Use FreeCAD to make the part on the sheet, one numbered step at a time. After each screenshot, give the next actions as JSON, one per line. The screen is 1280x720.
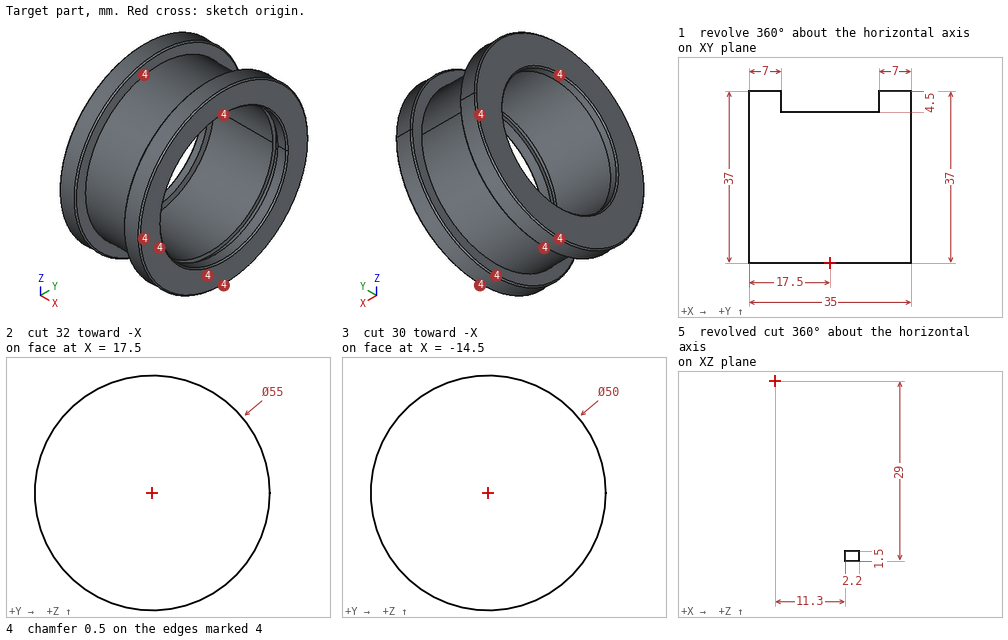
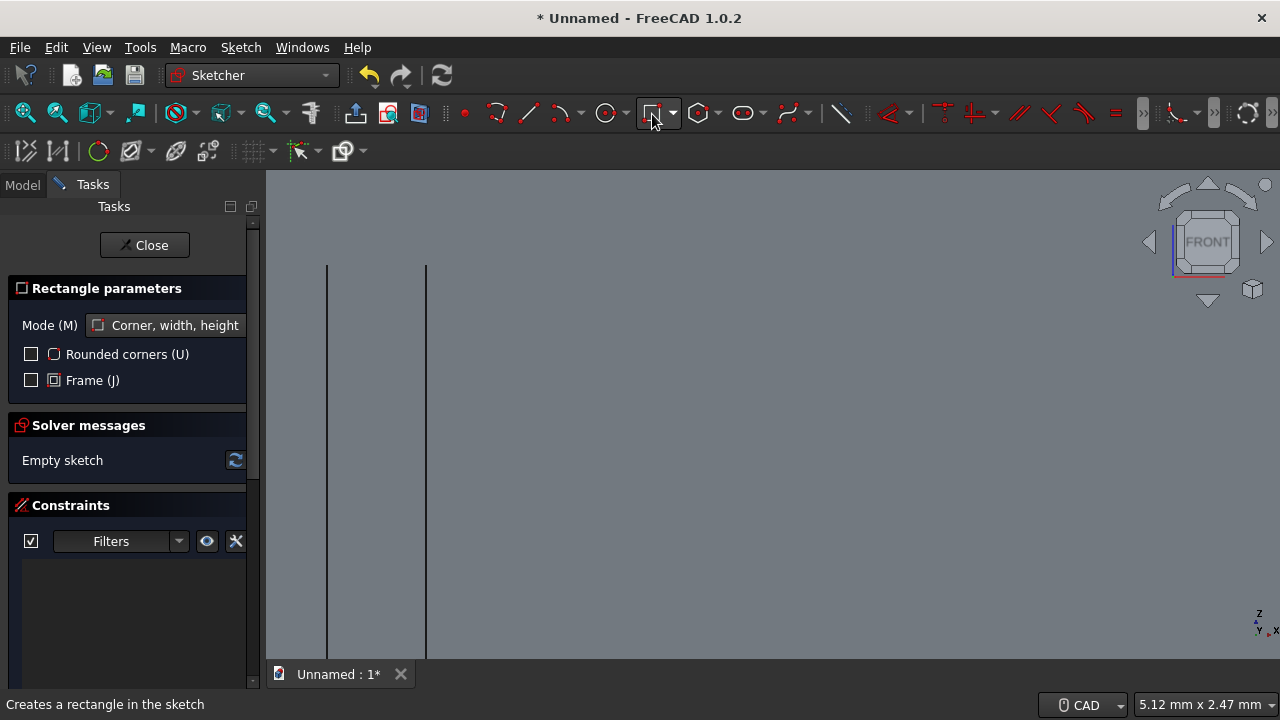
{"action": "left_click", "coordinate": [486, 265]}
{"action": "left_click", "coordinate": [922, 562]}
{"action": "key", "text": "Escape"}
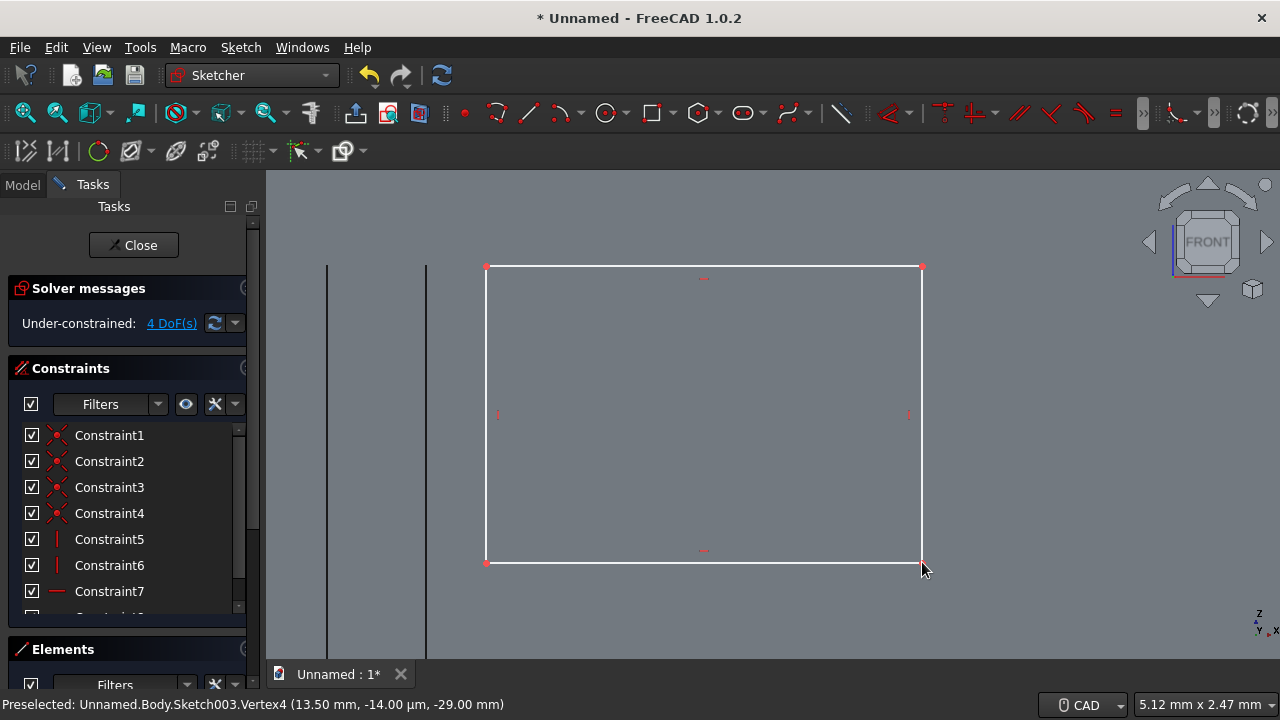
{"action": "left_click", "coordinate": [888, 114]}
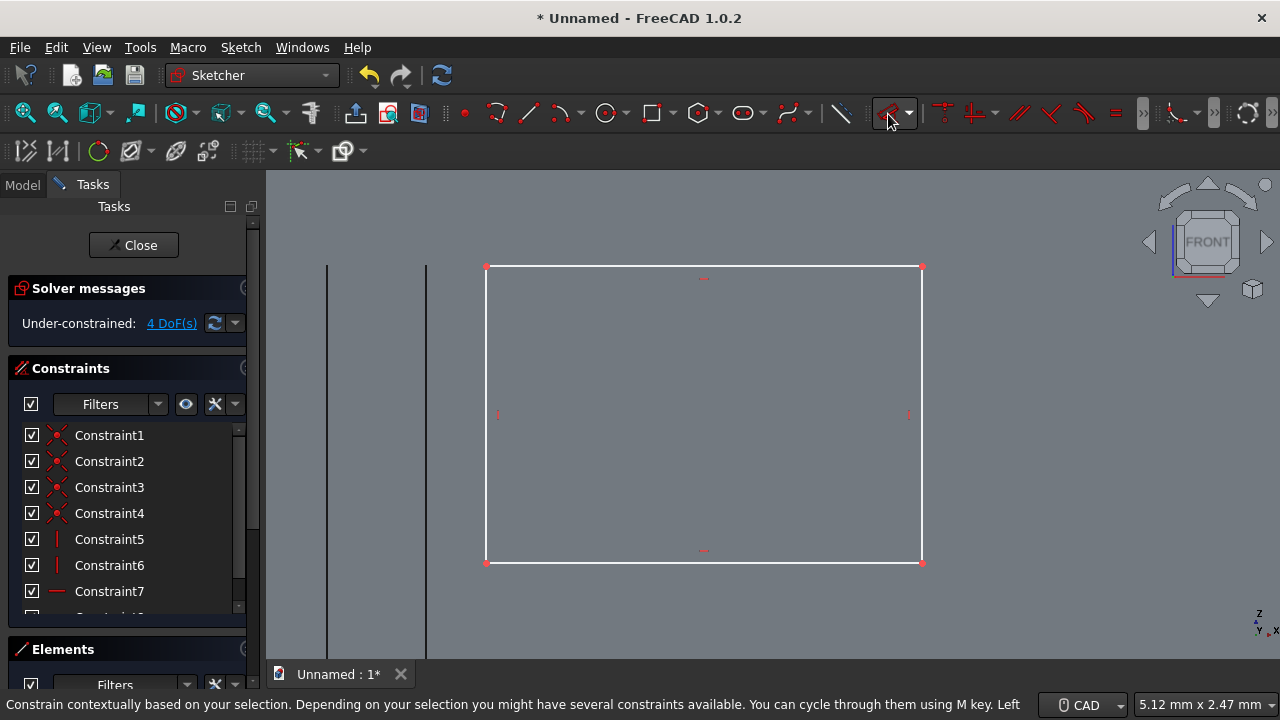
{"action": "left_click", "coordinate": [486, 355]}
{"action": "left_click", "coordinate": [452, 414]}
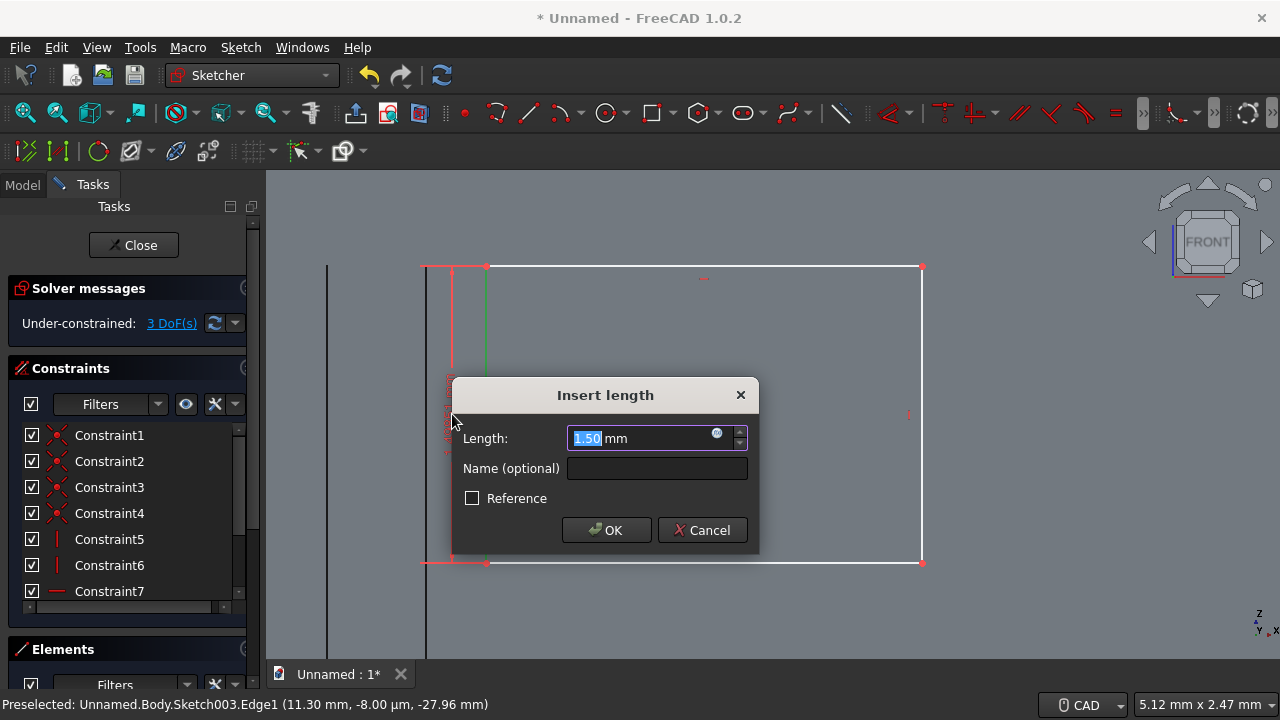
{"action": "type", "text": "1.5"}
{"action": "key", "text": "Return"}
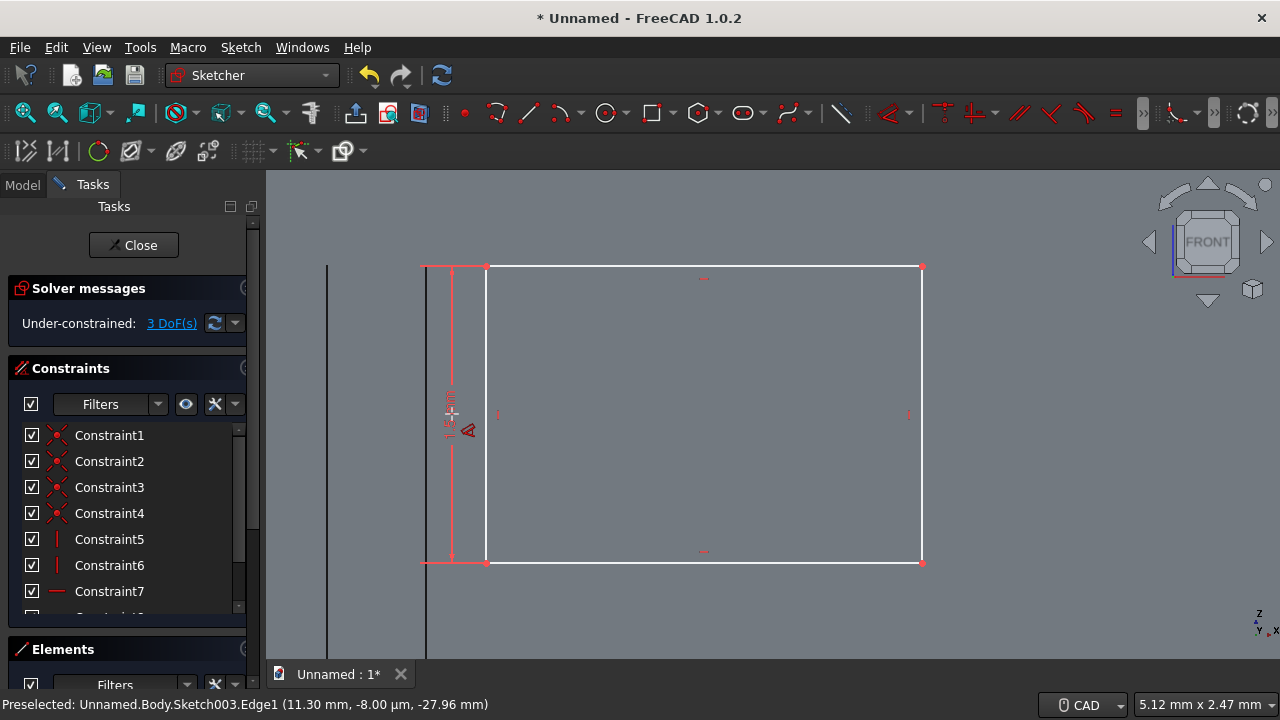
{"action": "left_click", "coordinate": [617, 563]}
{"action": "left_click", "coordinate": [704, 597]}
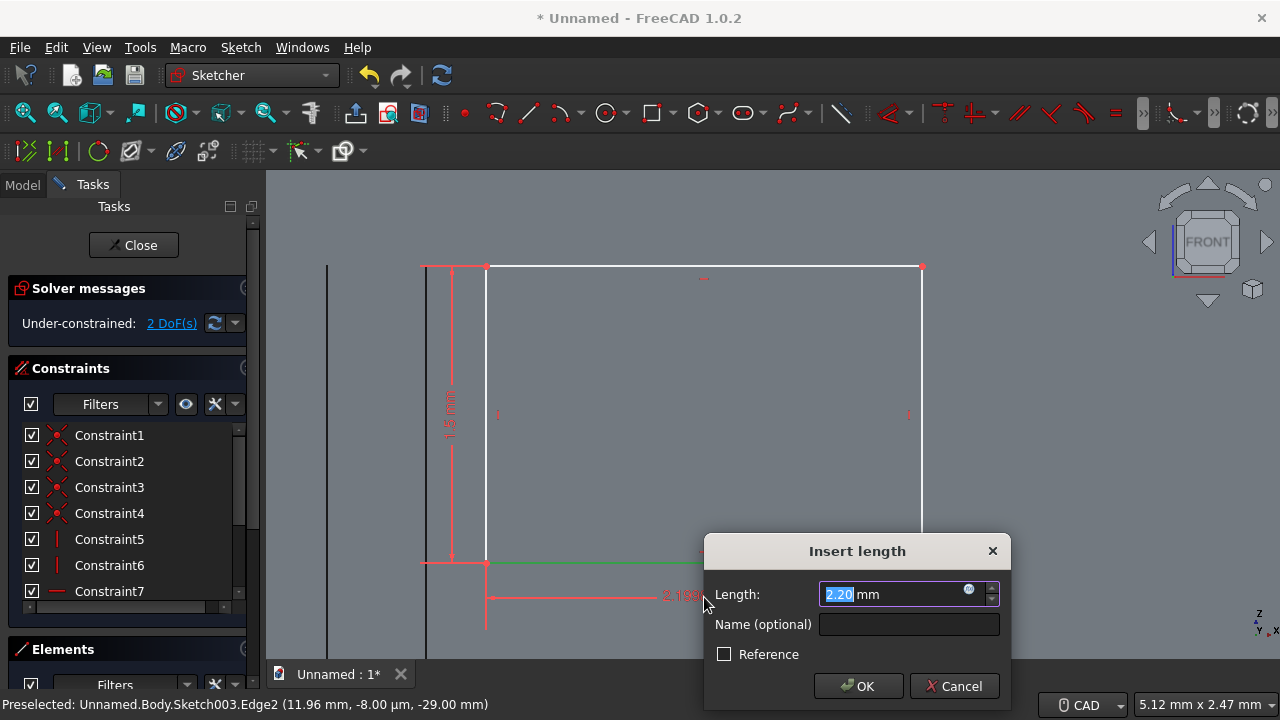
{"action": "type", "text": "2.2"}
{"action": "key", "text": "Return"}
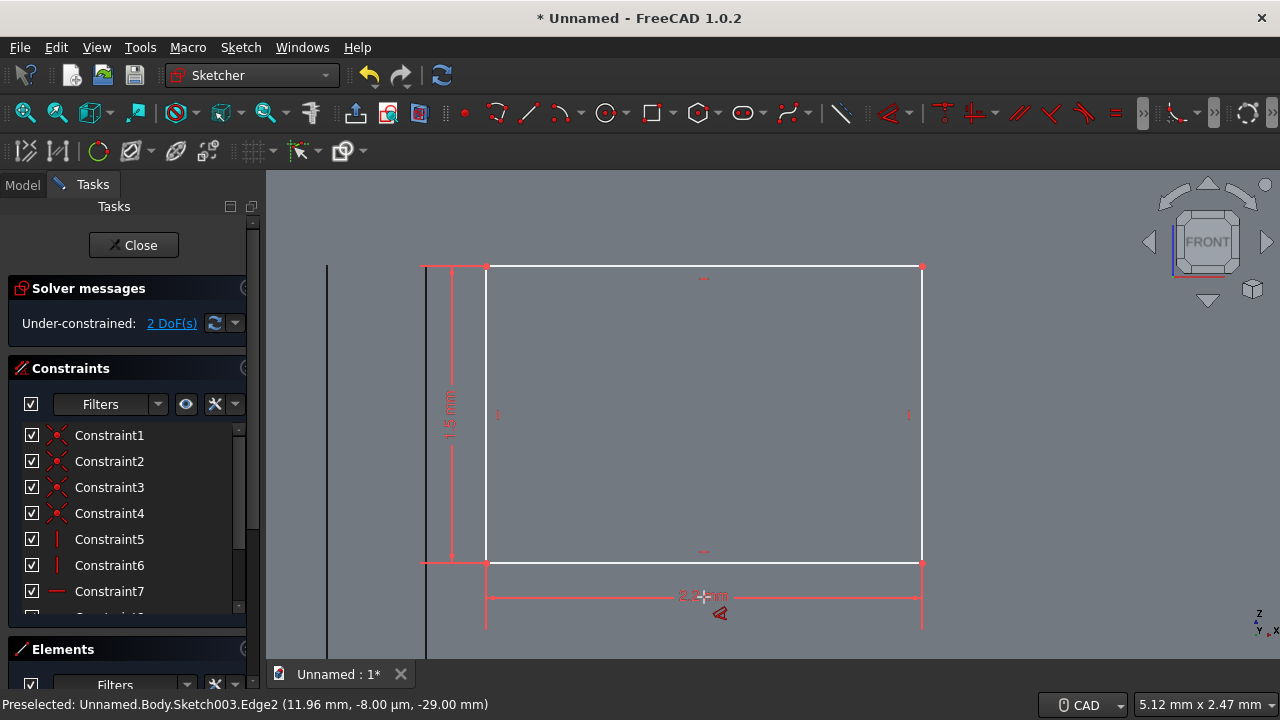
{"action": "left_click", "coordinate": [486, 563]}
{"action": "left_click", "coordinate": [520, 381]}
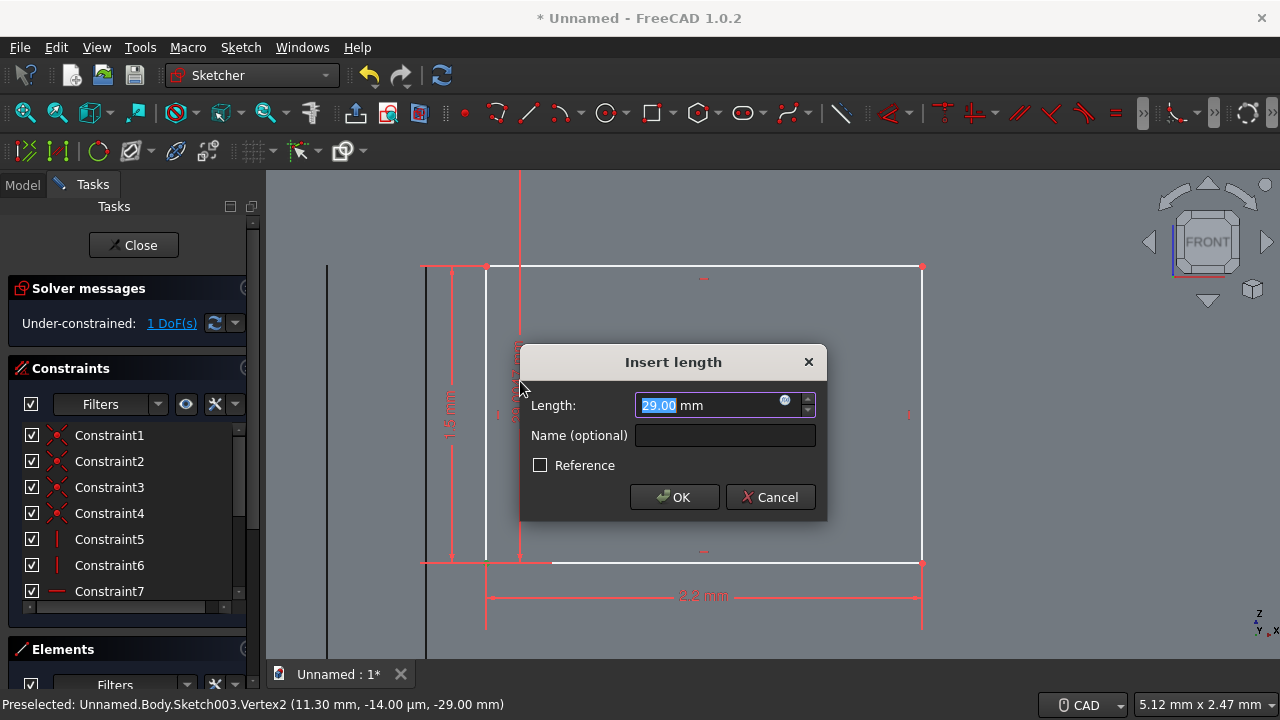
{"action": "type", "text": "29"}
{"action": "key", "text": "Return"}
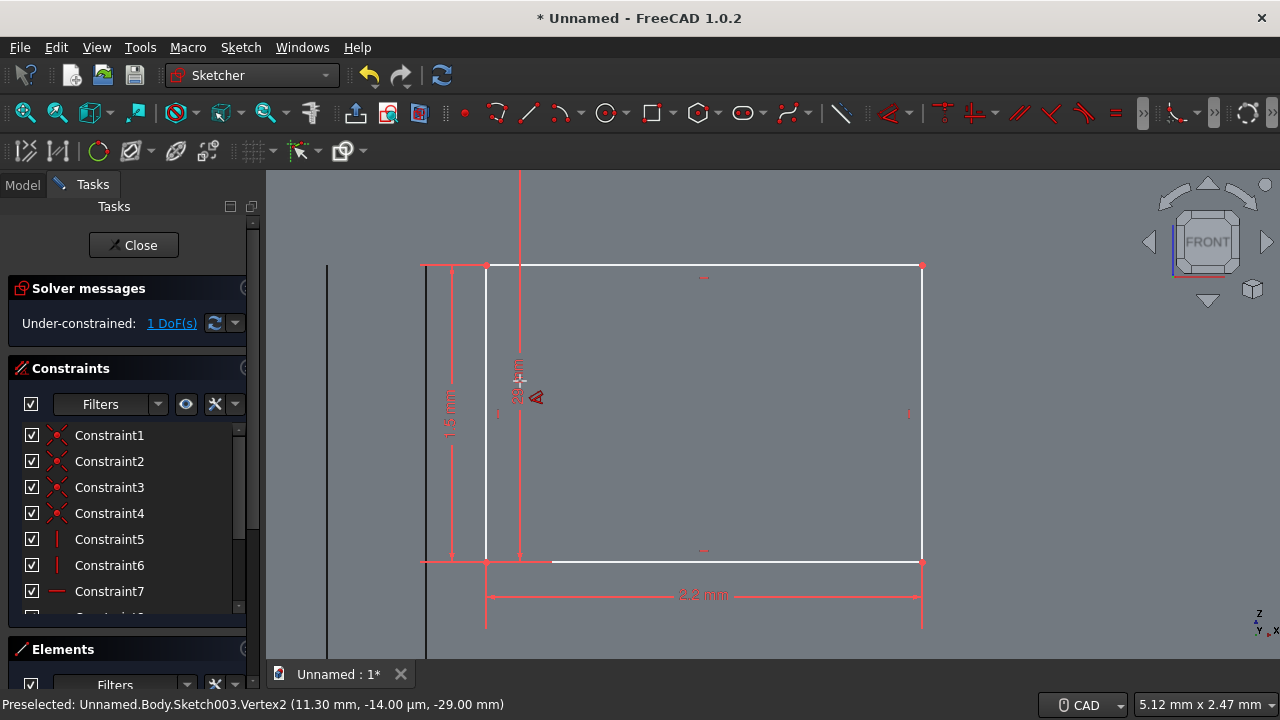
{"action": "left_click", "coordinate": [486, 265]}
{"action": "left_click", "coordinate": [390, 299]}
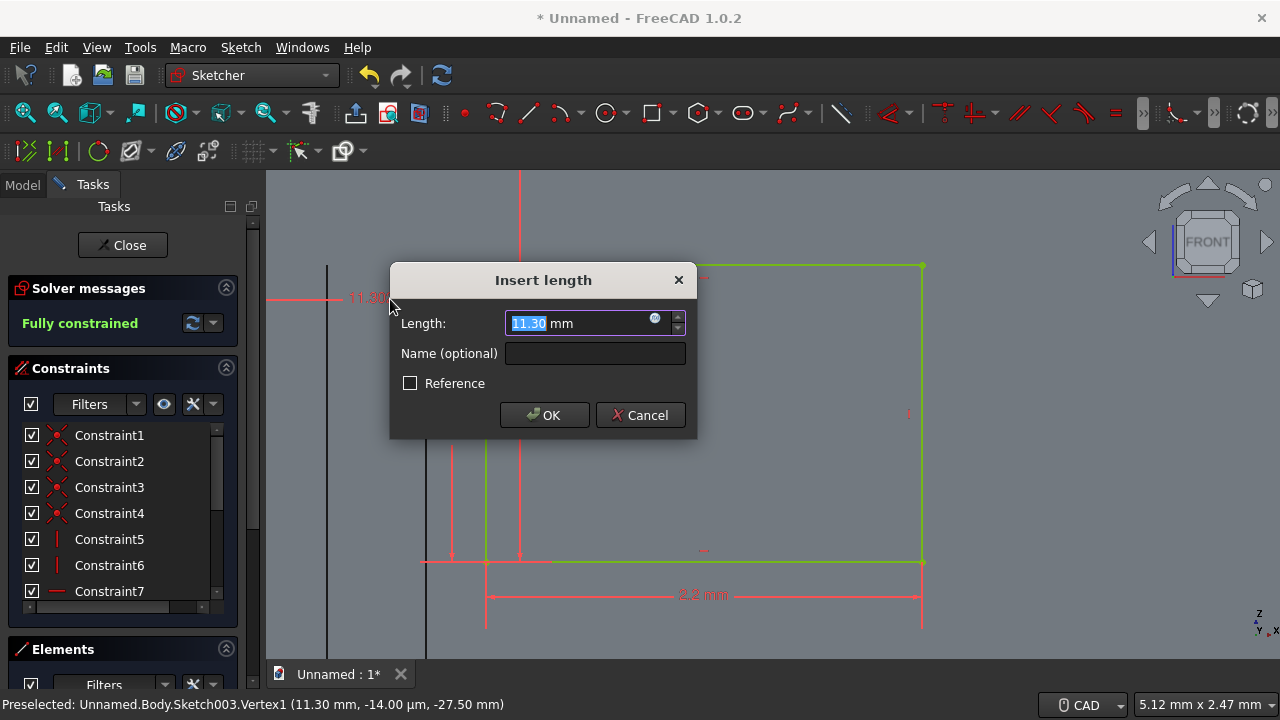
{"action": "type", "text": "11.3"}
{"action": "key", "text": "Return"}
{"action": "key", "text": "Escape"}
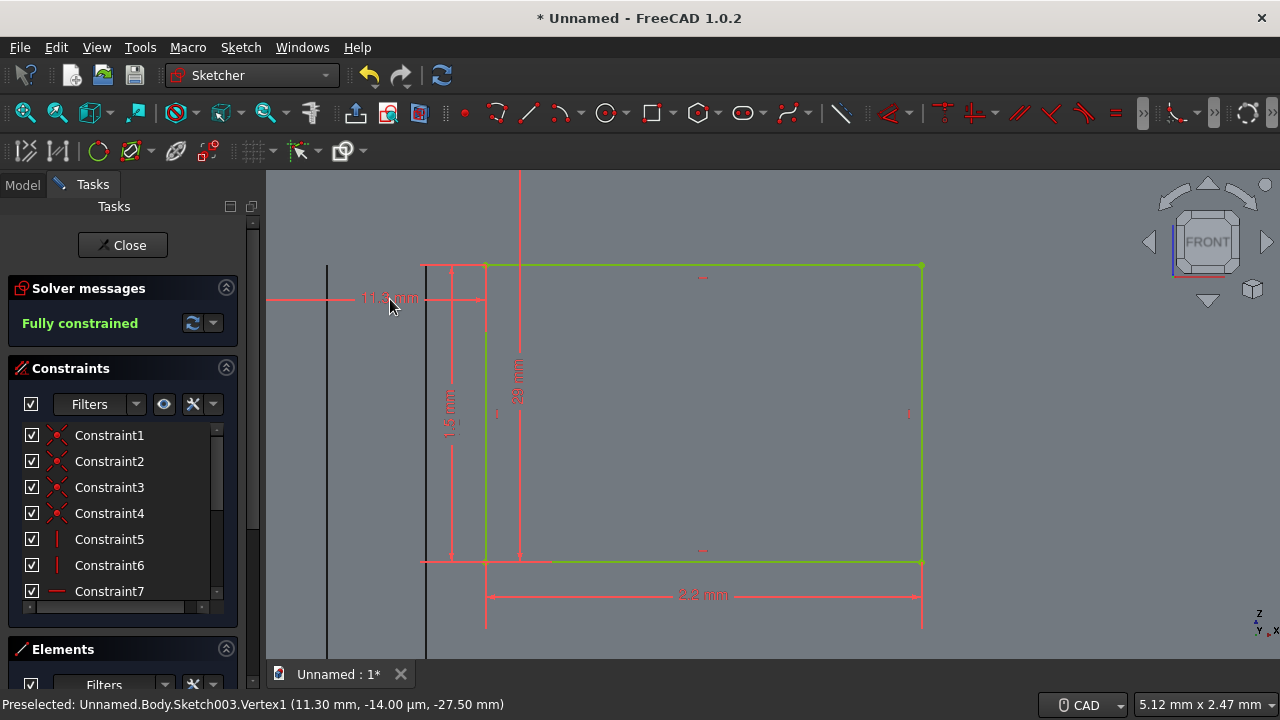
{"action": "left_click", "coordinate": [123, 245]}